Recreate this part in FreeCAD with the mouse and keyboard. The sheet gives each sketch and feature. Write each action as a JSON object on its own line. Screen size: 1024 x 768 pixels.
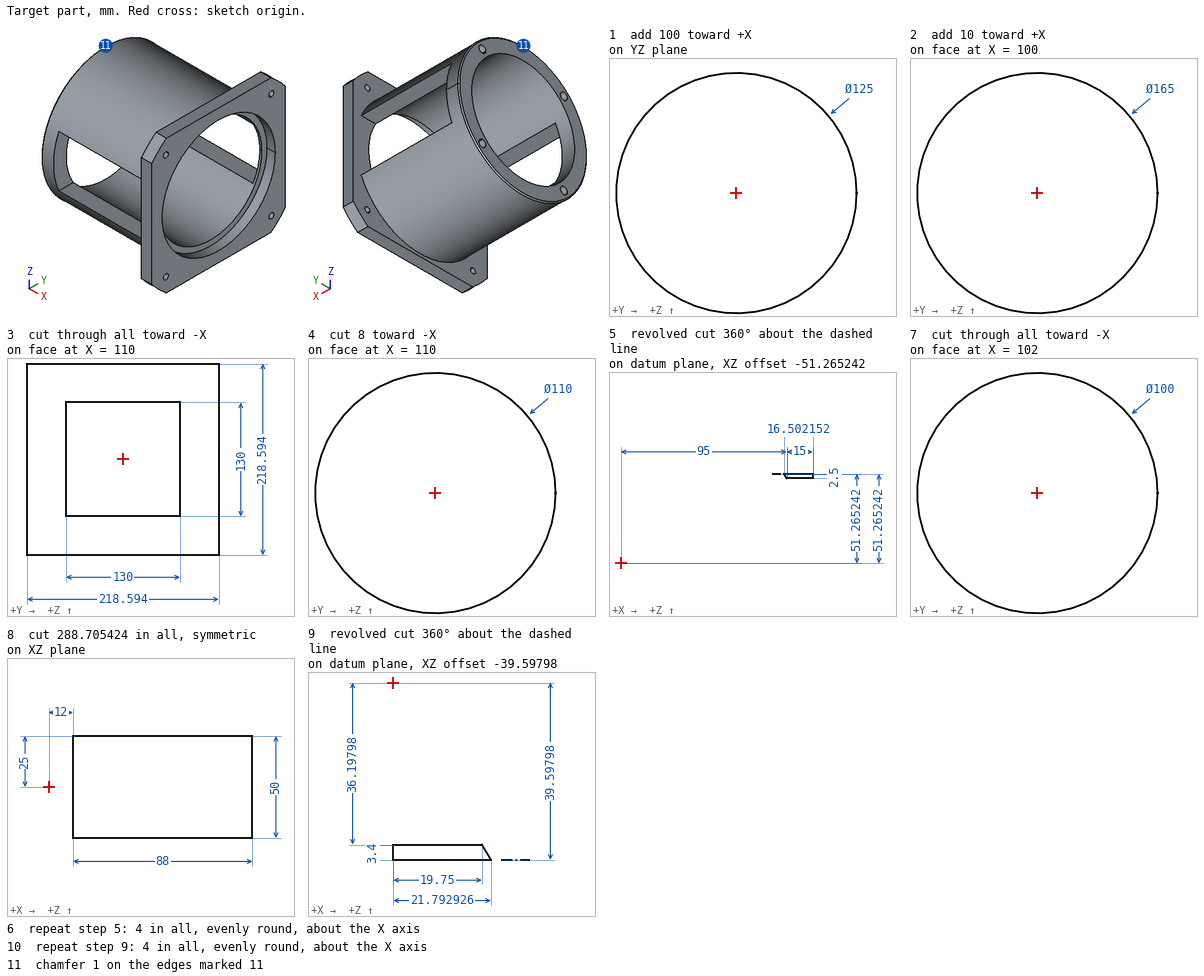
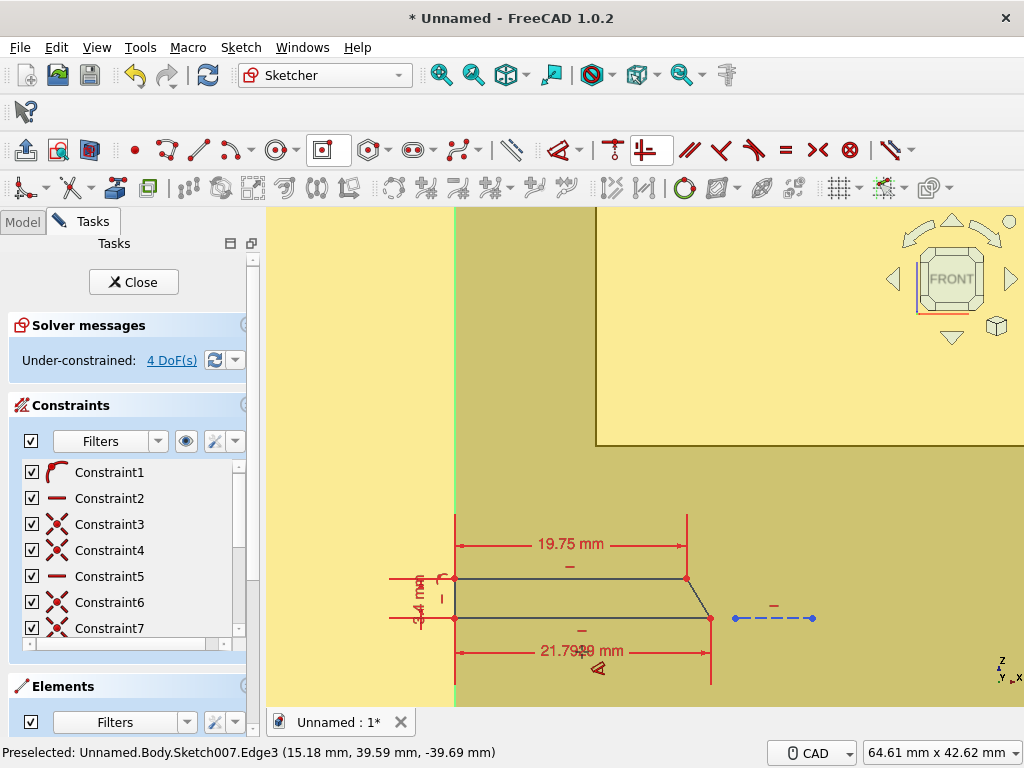
{"action": "left_click", "coordinate": [455, 579]}
{"action": "left_click", "coordinate": [421, 407]}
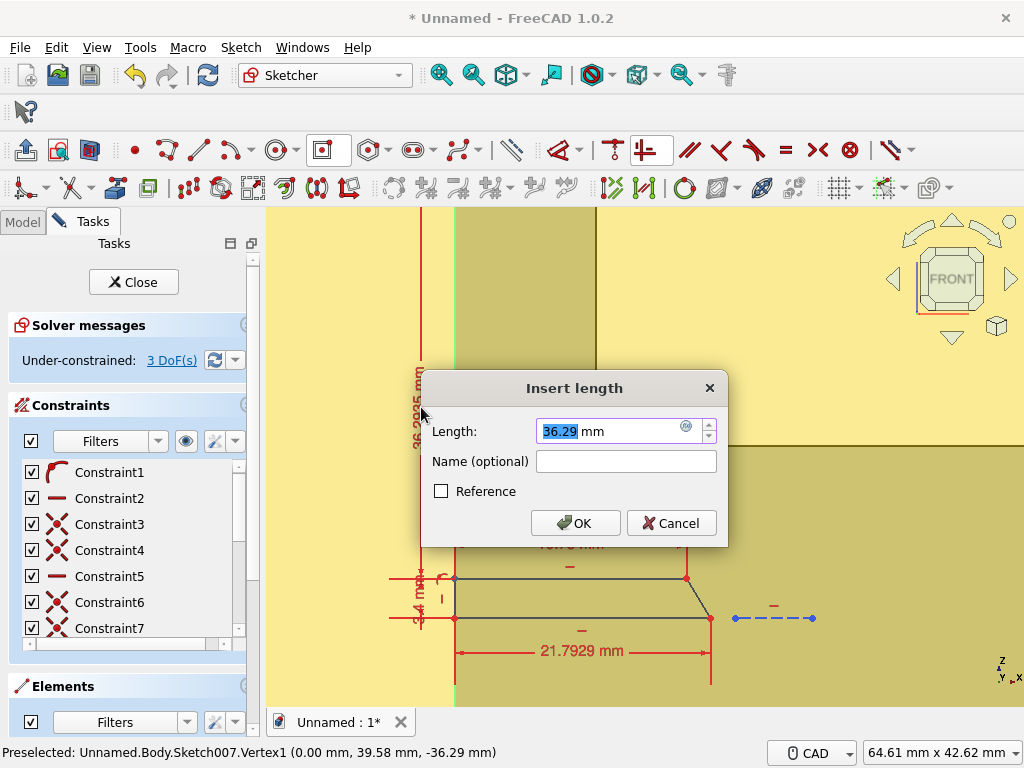
{"action": "type", "text": "36.19798"}
{"action": "key", "text": "Return"}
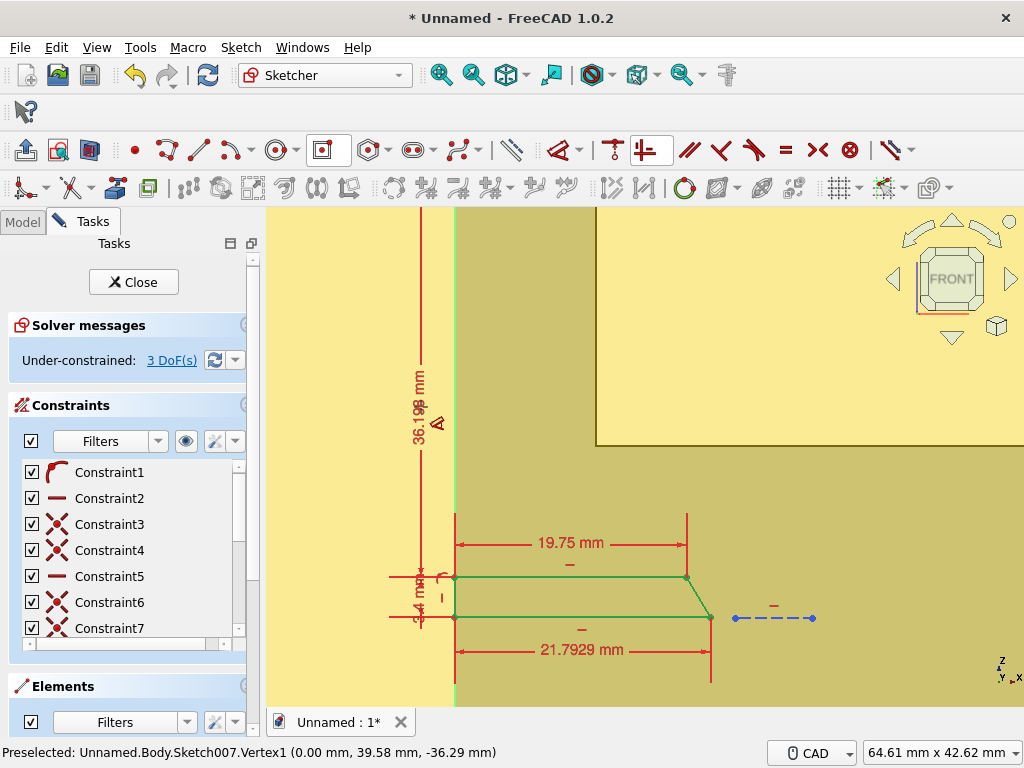
{"action": "left_click", "coordinate": [735, 618]}
{"action": "left_click", "coordinate": [421, 339]}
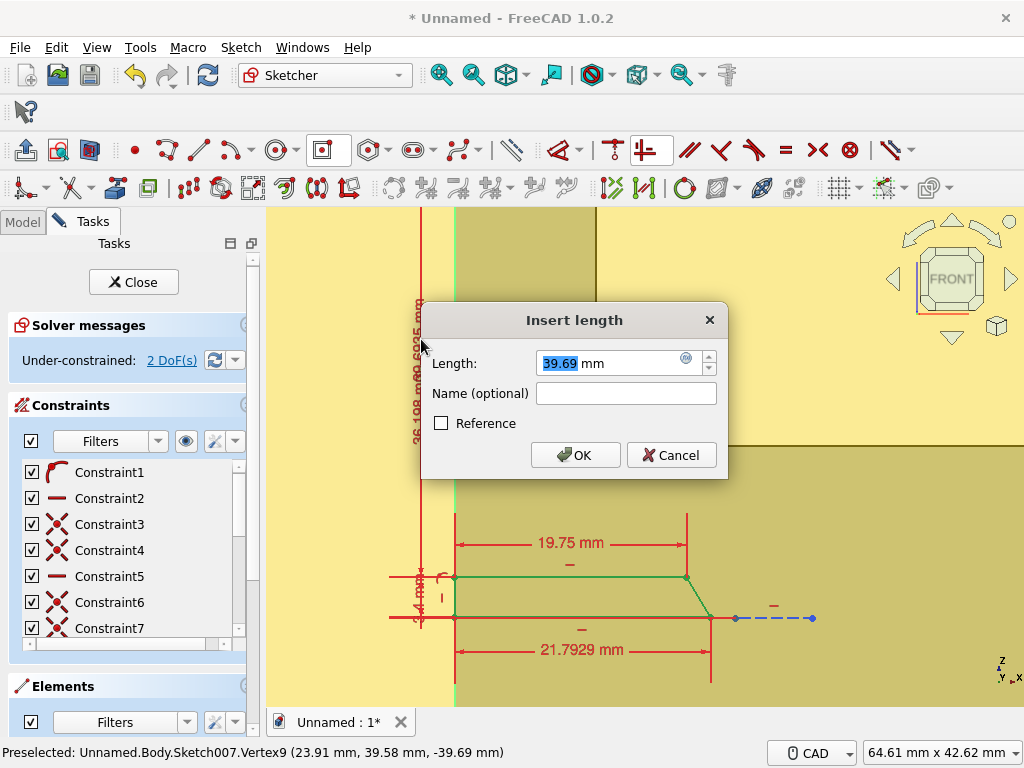
{"action": "type", "text": "39.59798"}
{"action": "key", "text": "Return"}
{"action": "key", "text": "Escape"}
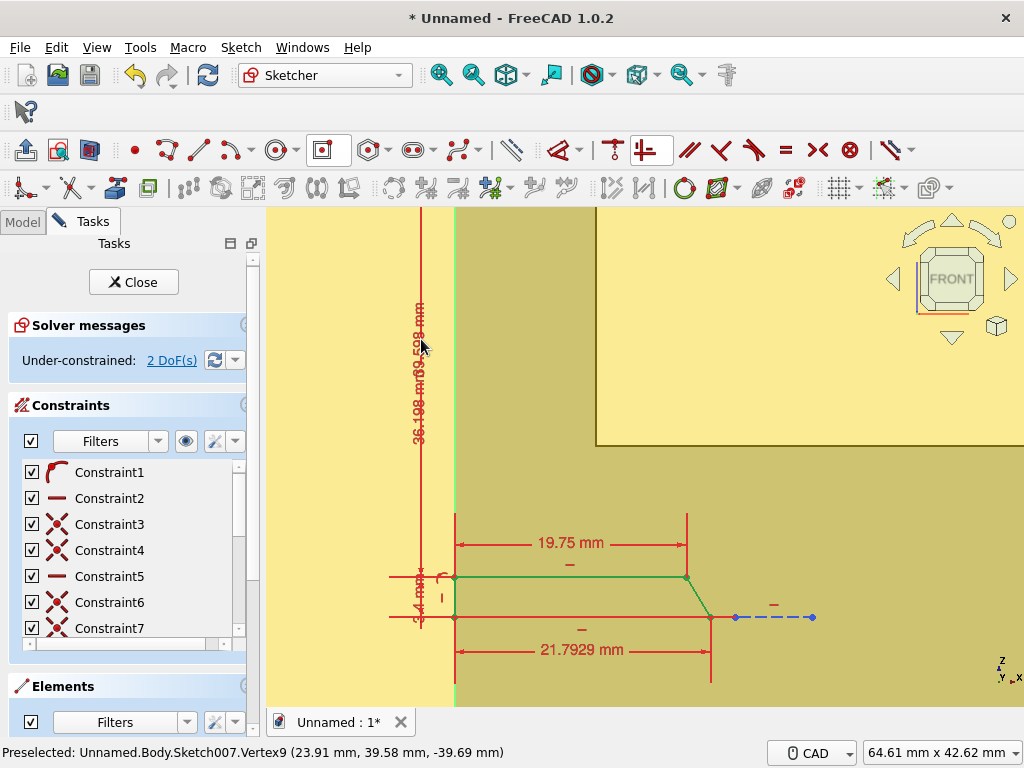
{"action": "left_click", "coordinate": [134, 282]}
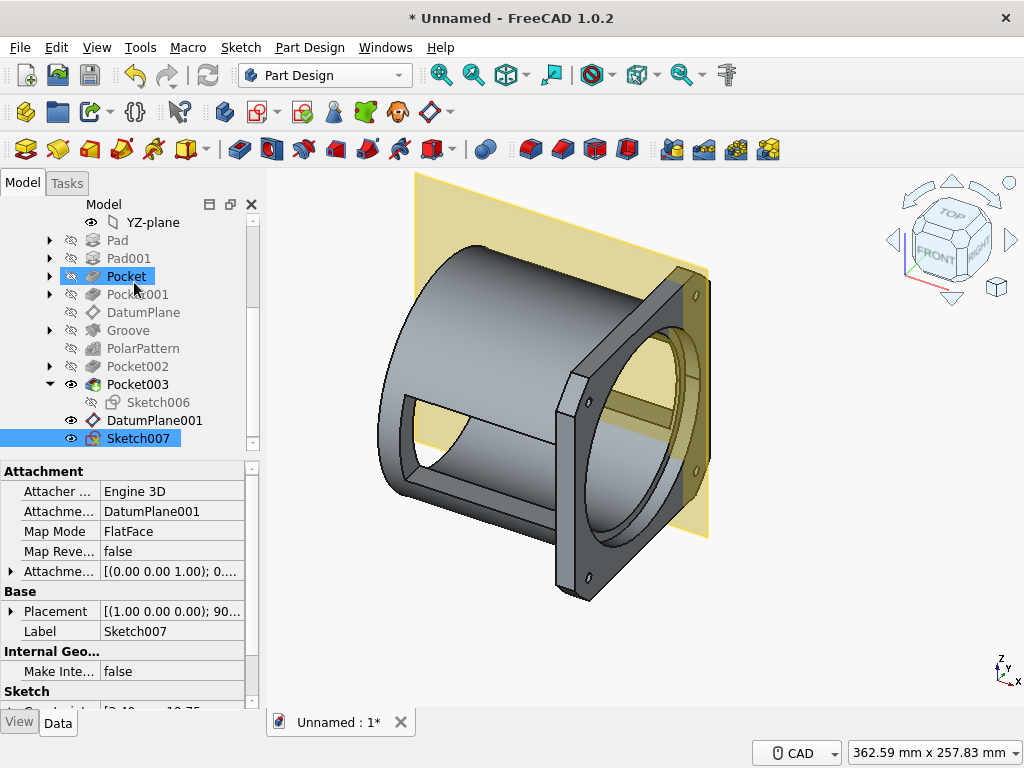
{"action": "left_click", "coordinate": [304, 150]}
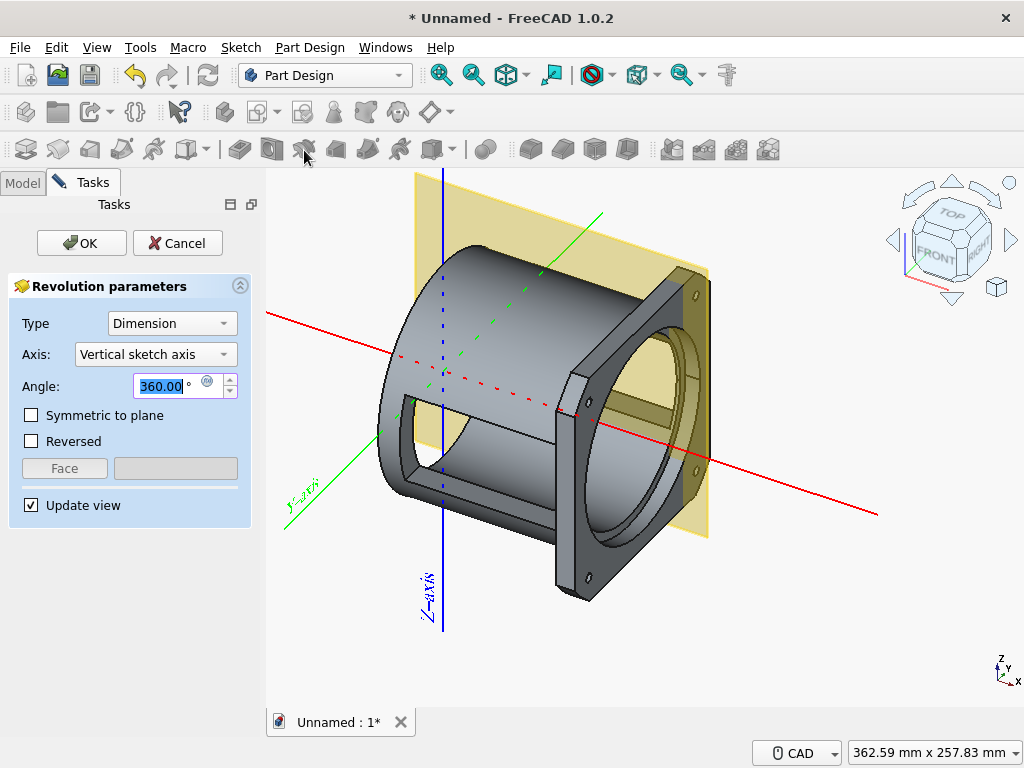
{"action": "left_click", "coordinate": [156, 354]}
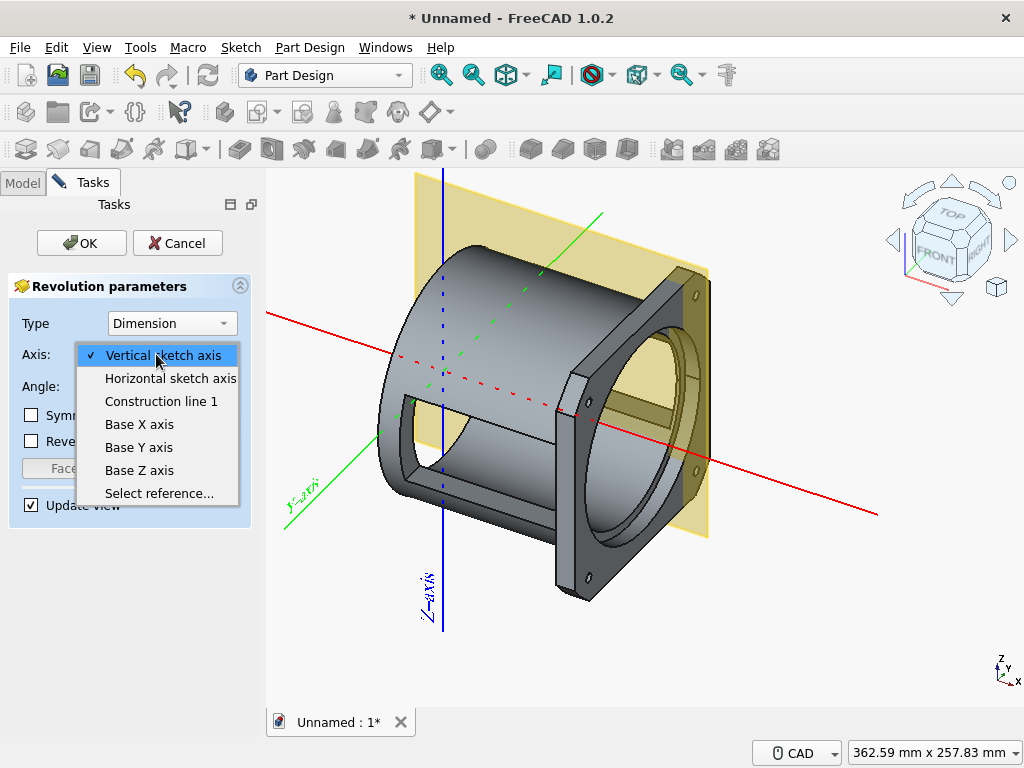
{"action": "left_click", "coordinate": [156, 402]}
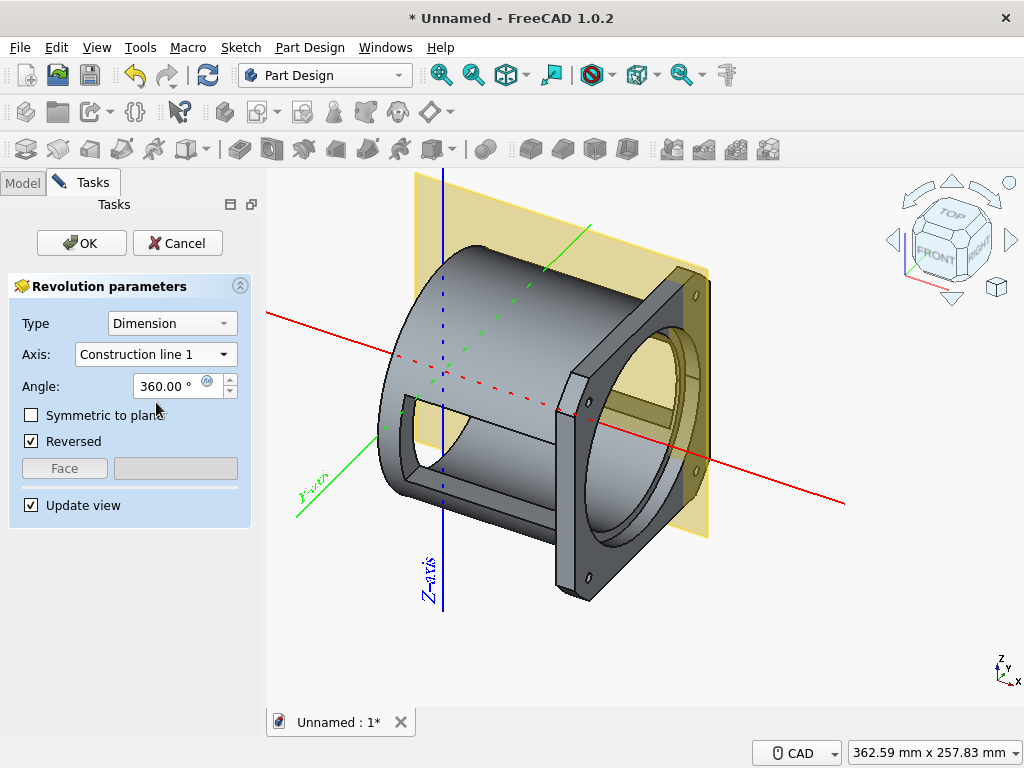
{"action": "left_click", "coordinate": [82, 243]}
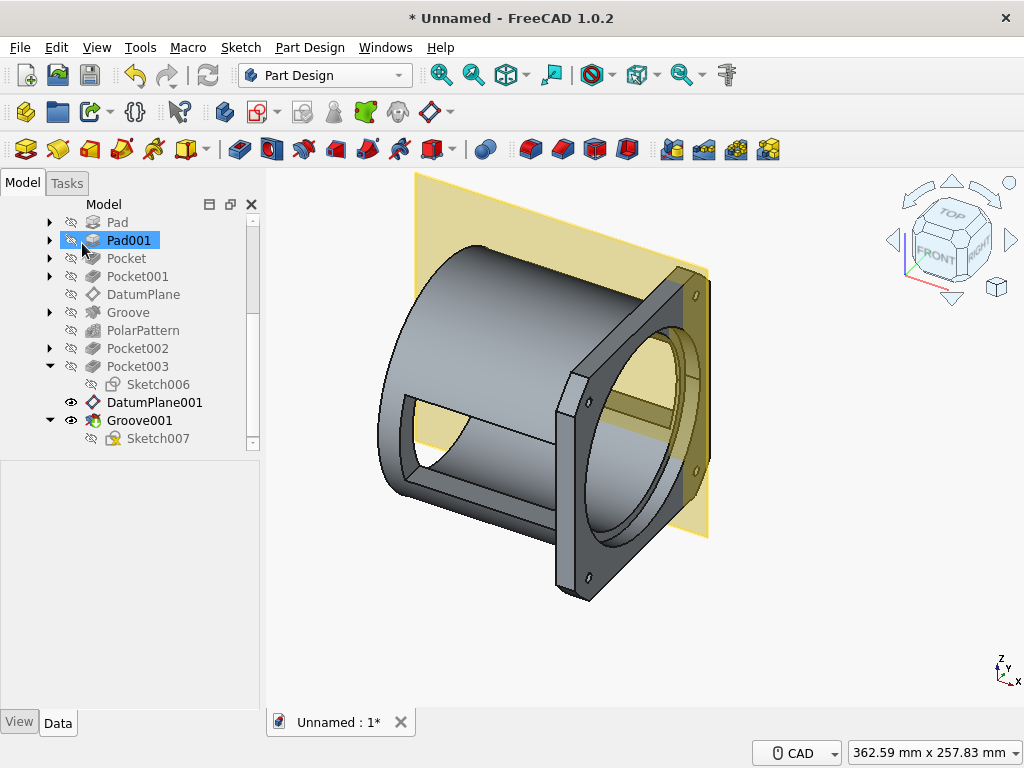
{"action": "left_click", "coordinate": [116, 402]}
{"action": "key", "text": "space"}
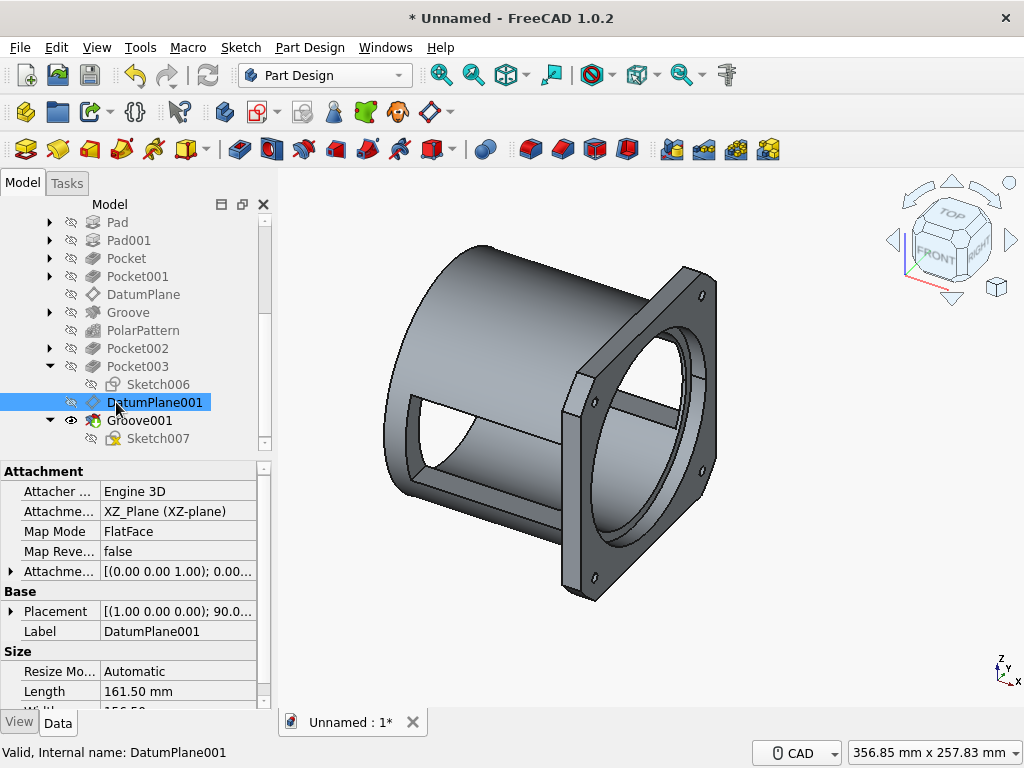
{"action": "left_click", "coordinate": [116, 420]}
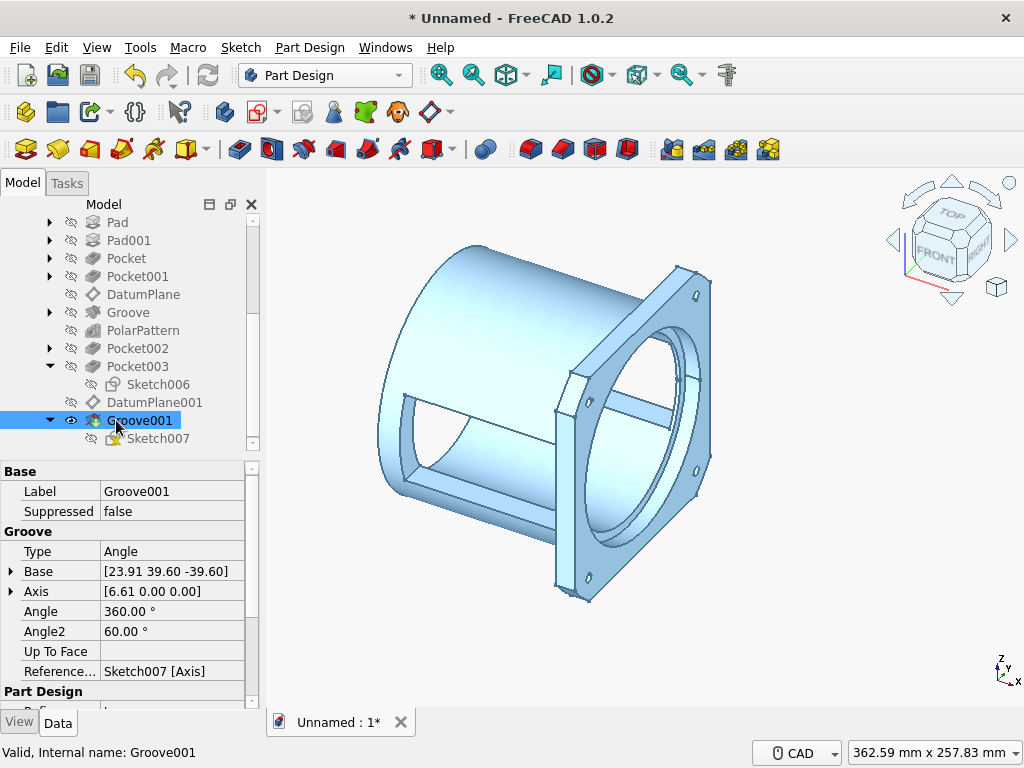
{"action": "left_click", "coordinate": [736, 150]}